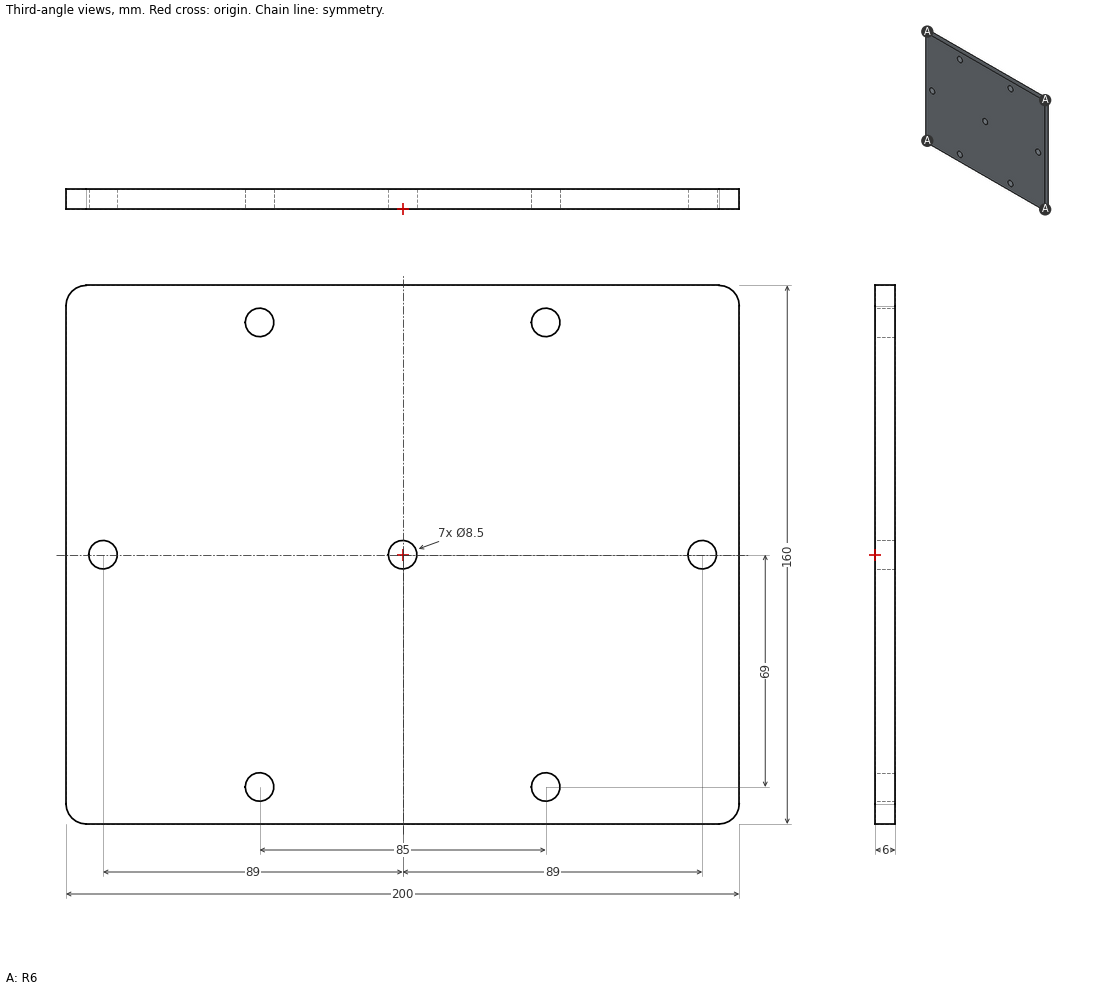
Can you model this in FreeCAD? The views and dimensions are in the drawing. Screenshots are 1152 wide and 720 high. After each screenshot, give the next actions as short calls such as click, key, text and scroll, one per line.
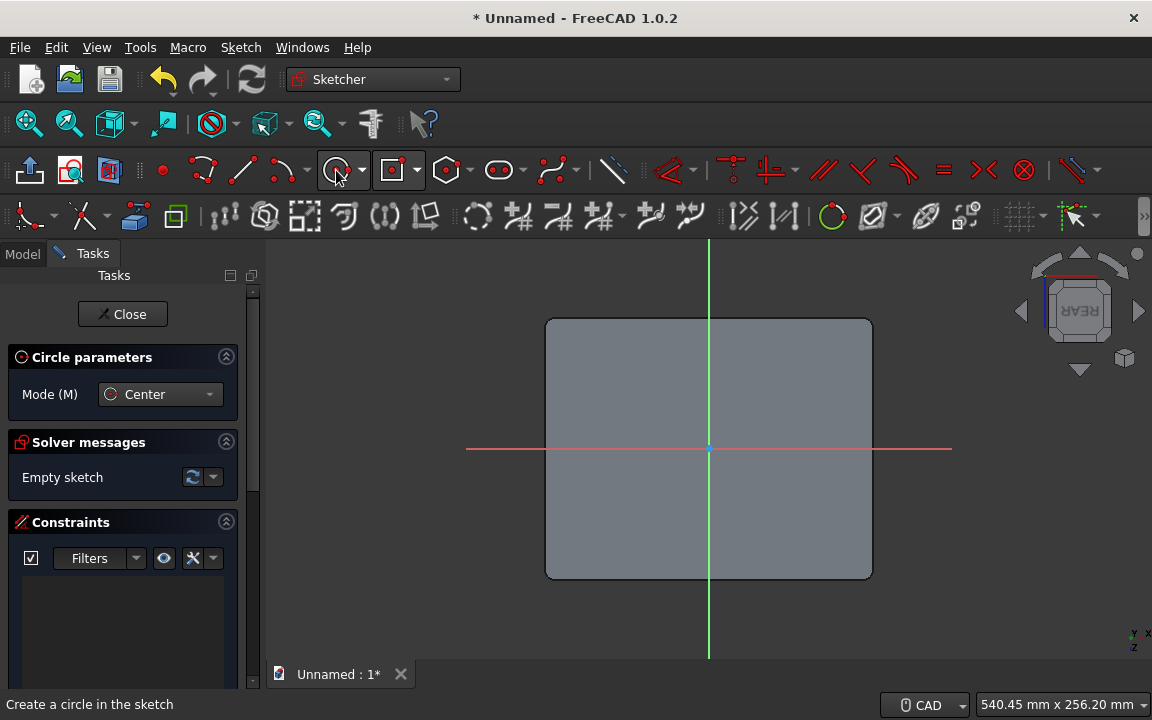
scroll(709, 449, up, 6)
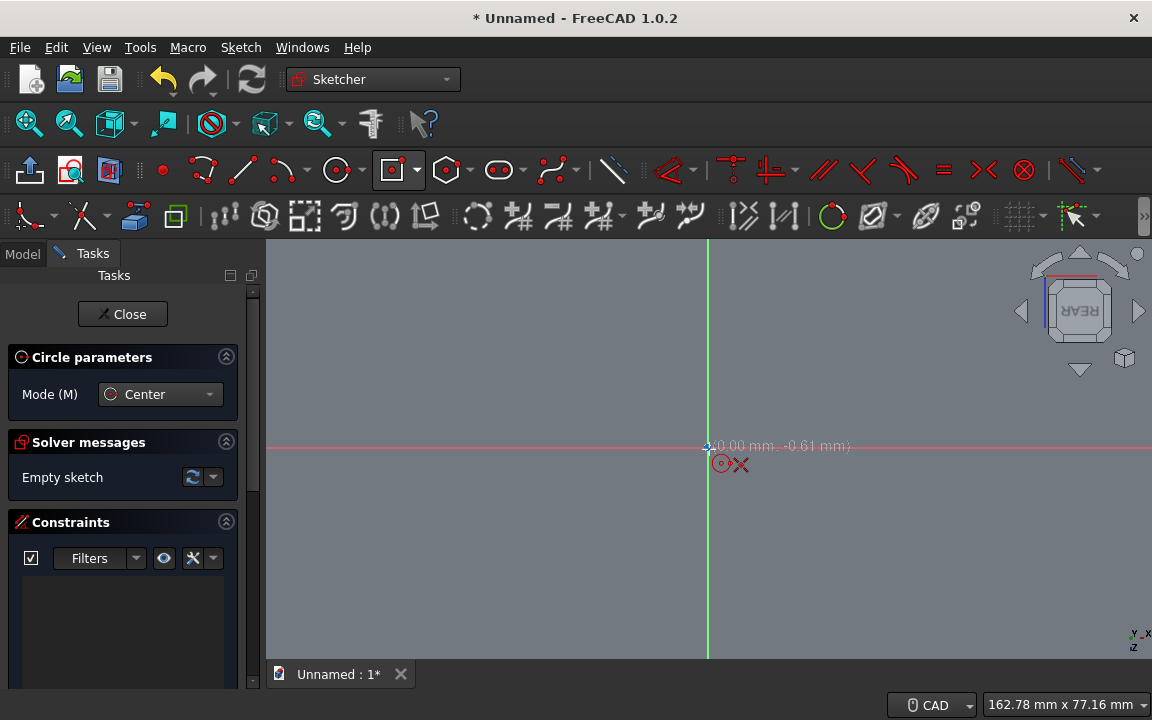
click(708, 448)
click(724, 431)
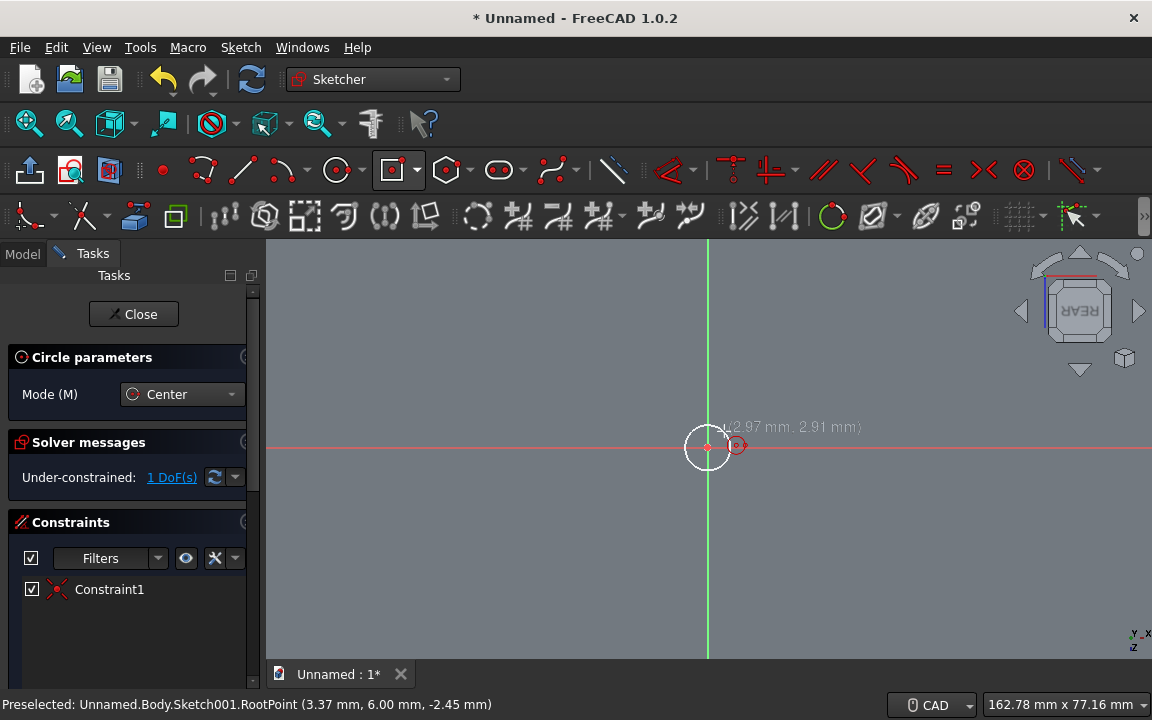
scroll(611, 450, down, 6)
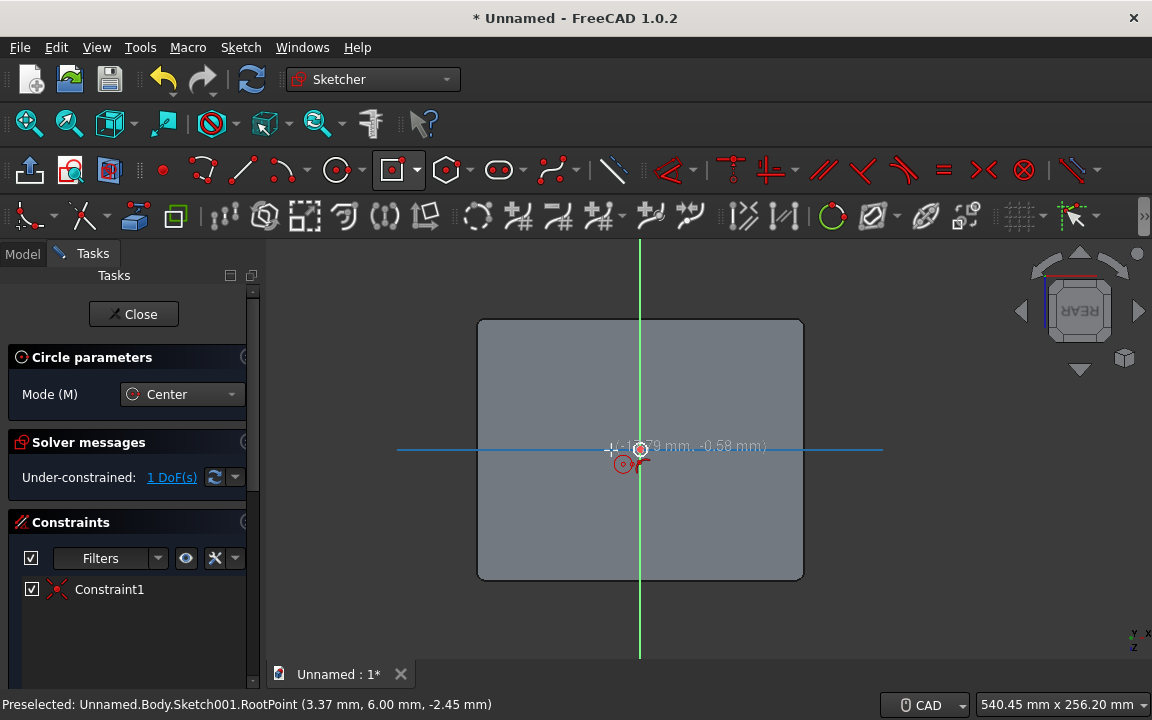
scroll(710, 337, up, 6)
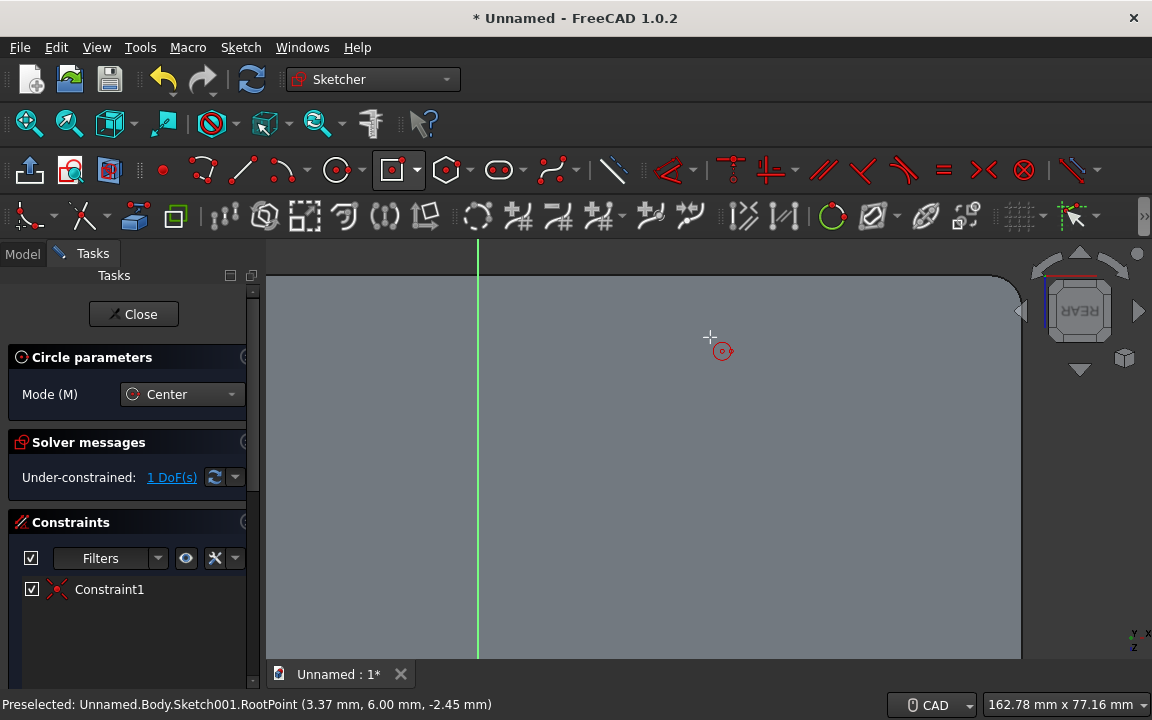
click(709, 335)
click(726, 319)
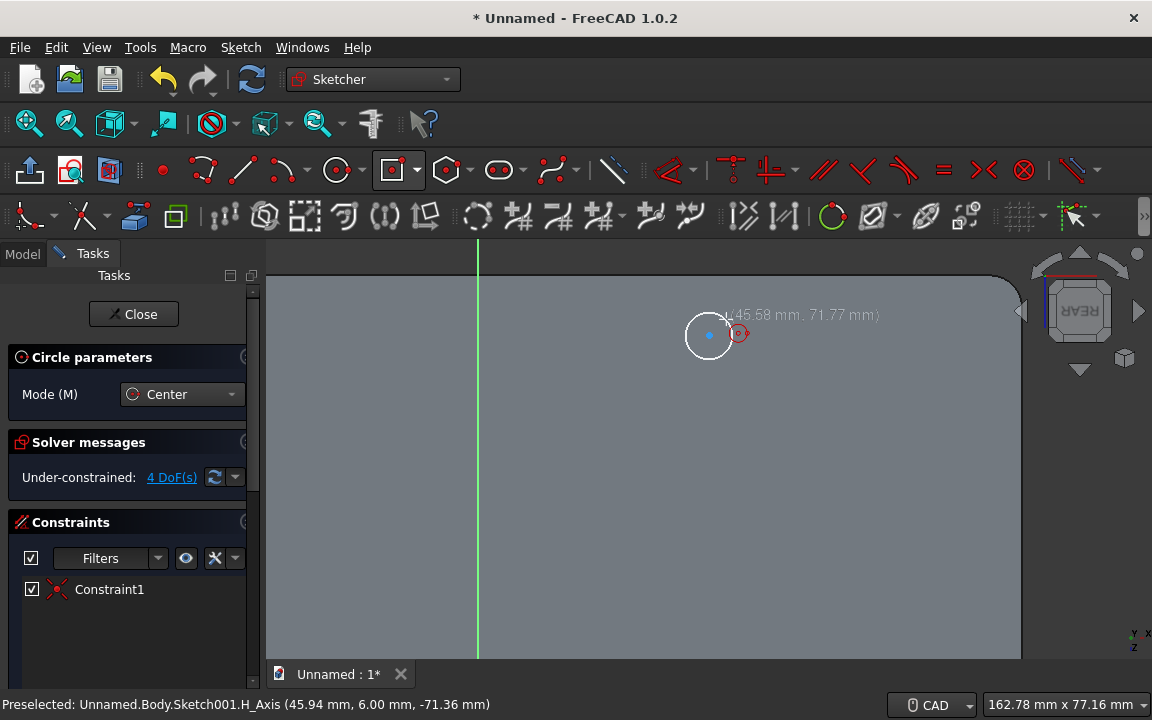
scroll(711, 336, down, 6)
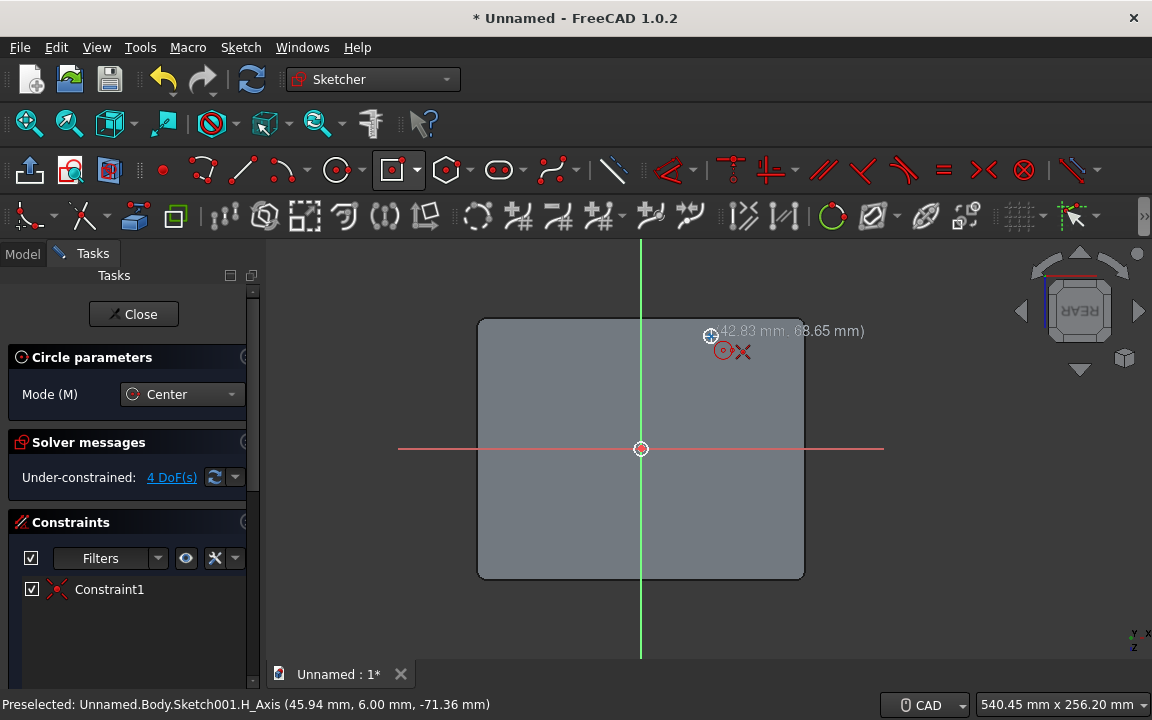
scroll(571, 336, up, 6)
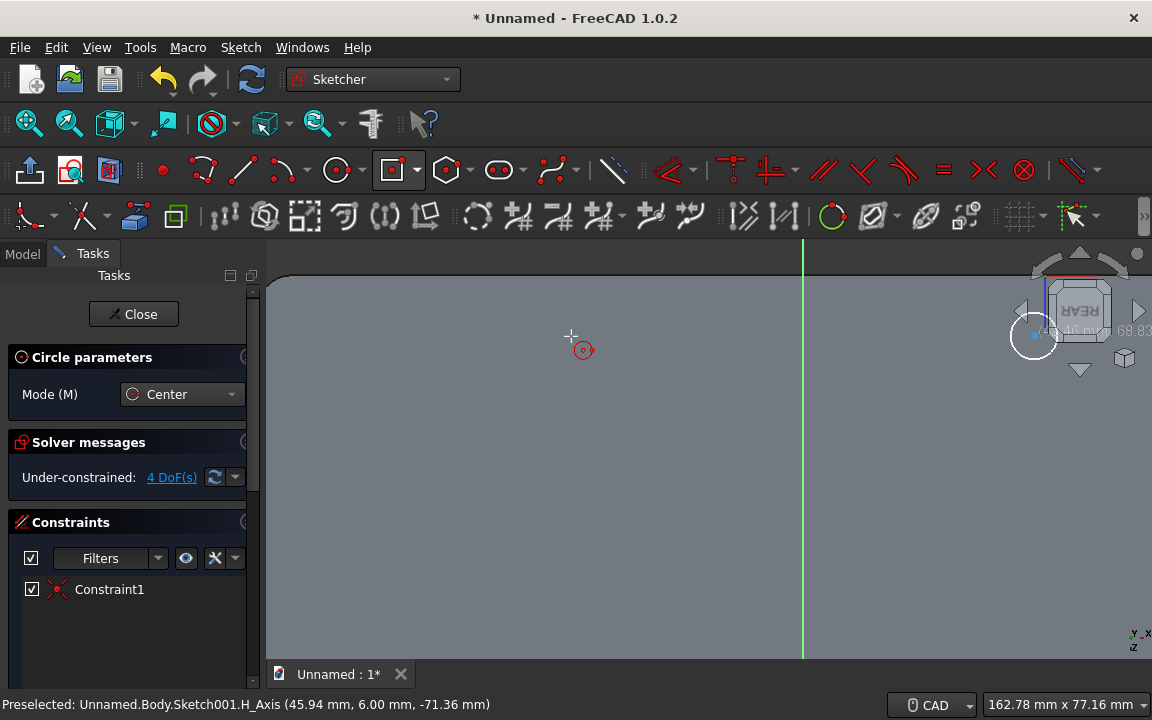
click(572, 335)
click(588, 319)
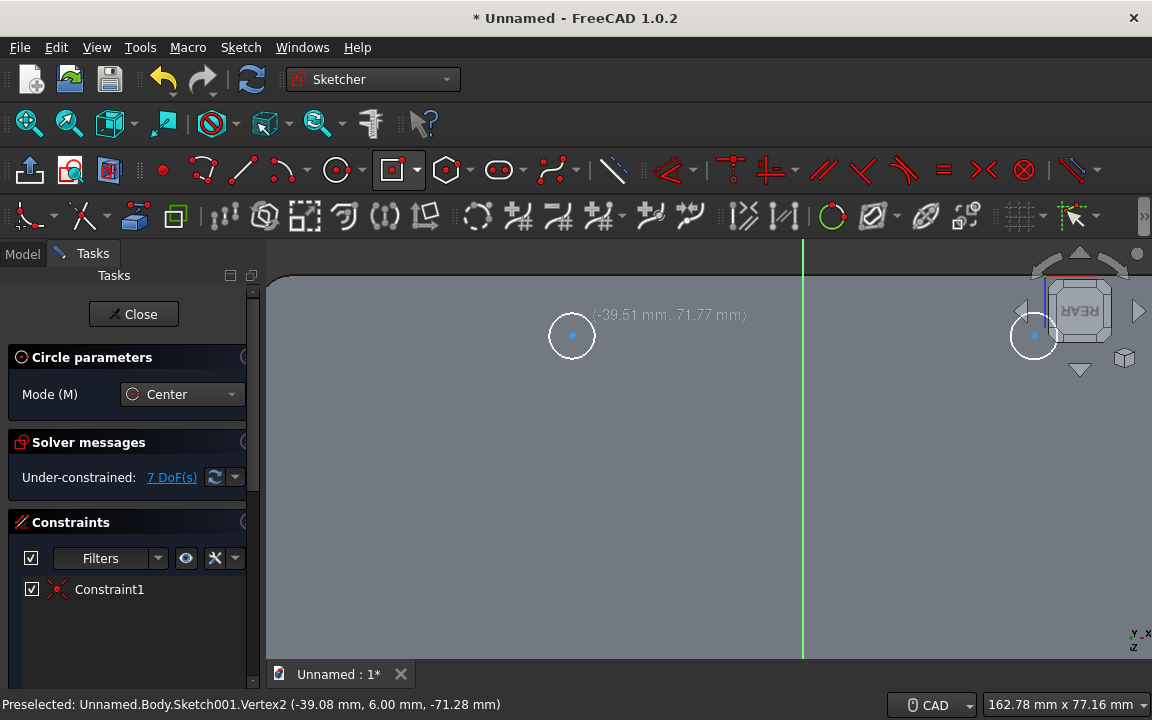
scroll(570, 336, down, 6)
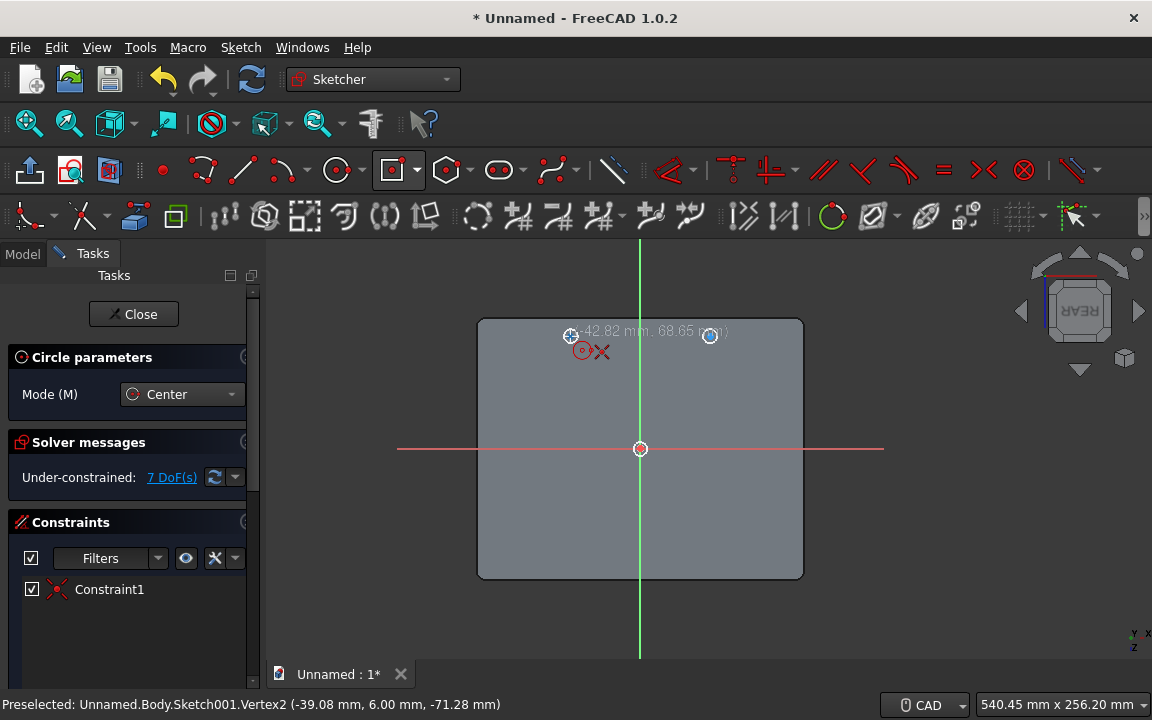
scroll(495, 449, up, 6)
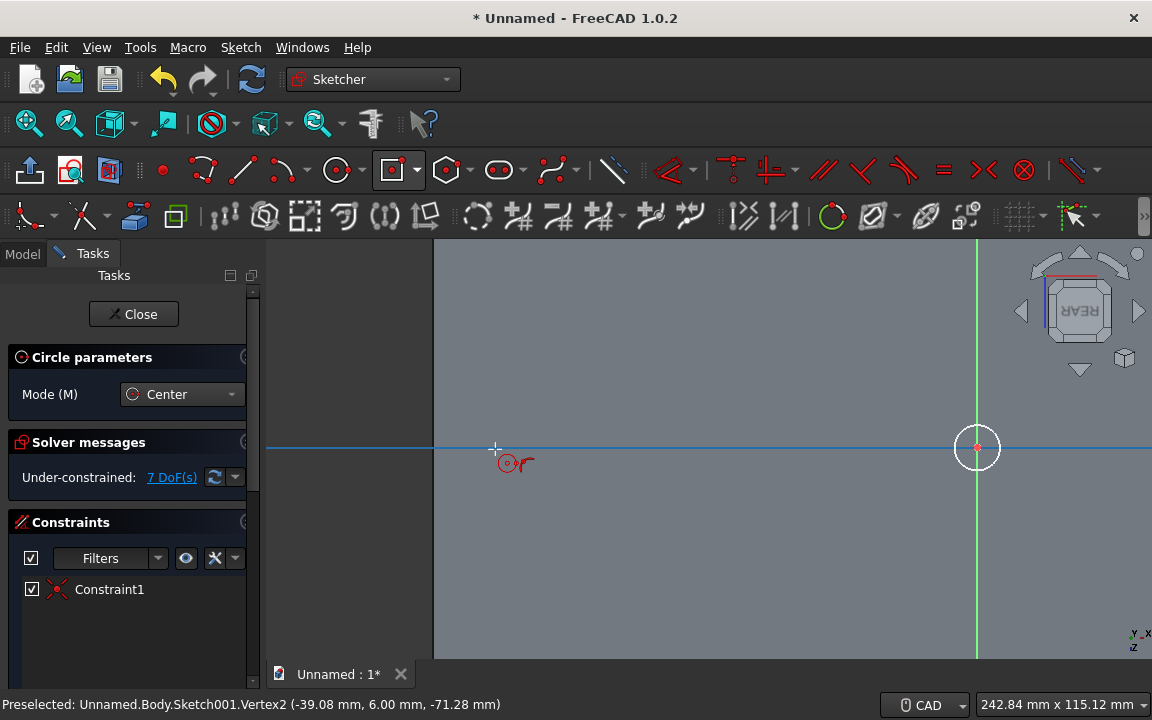
click(493, 448)
click(509, 431)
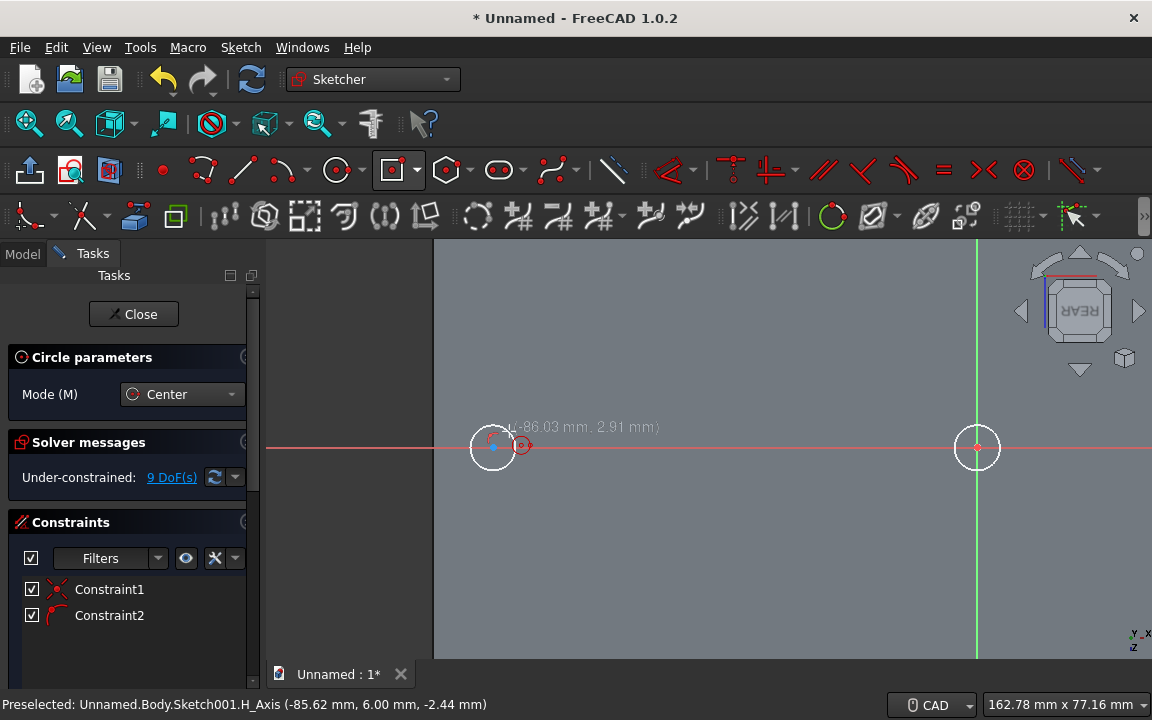
scroll(495, 450, down, 6)